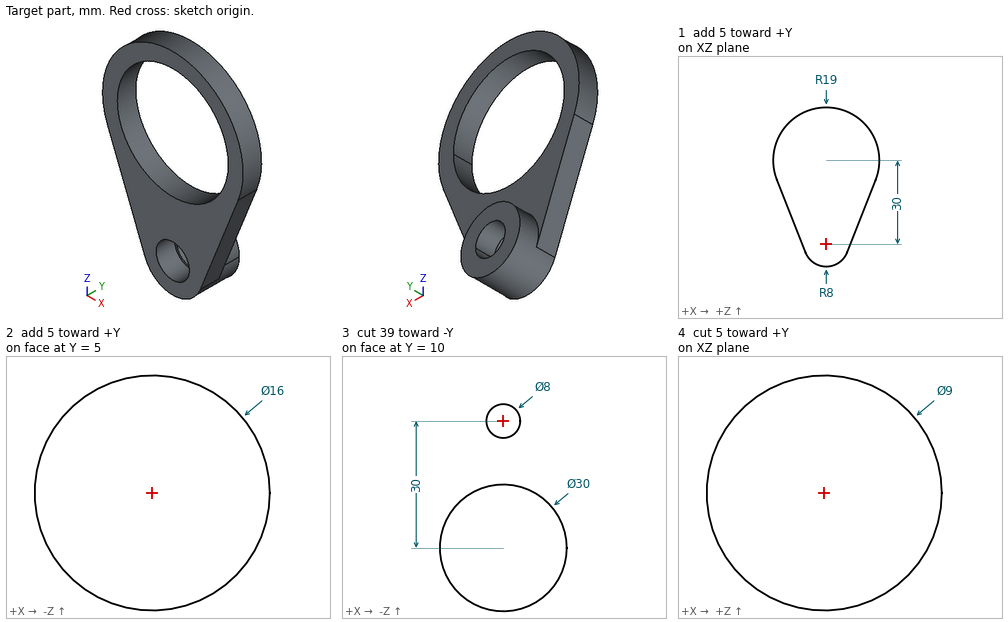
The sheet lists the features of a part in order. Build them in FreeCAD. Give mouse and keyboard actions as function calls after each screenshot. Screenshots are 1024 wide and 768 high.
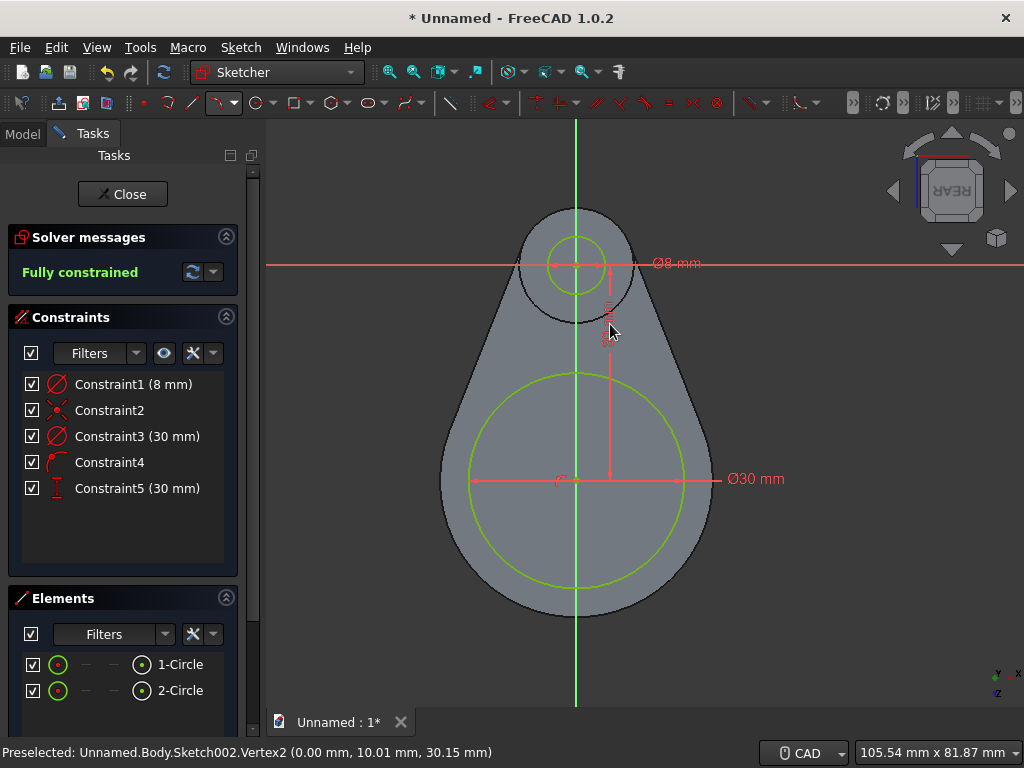
click(123, 194)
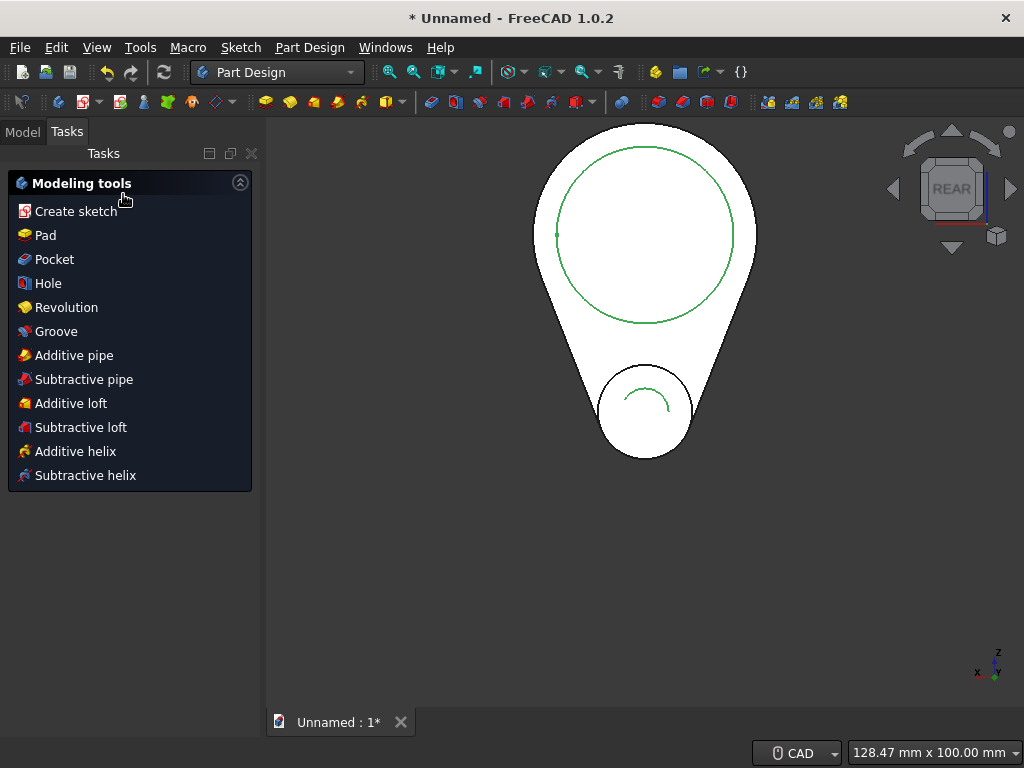
click(432, 102)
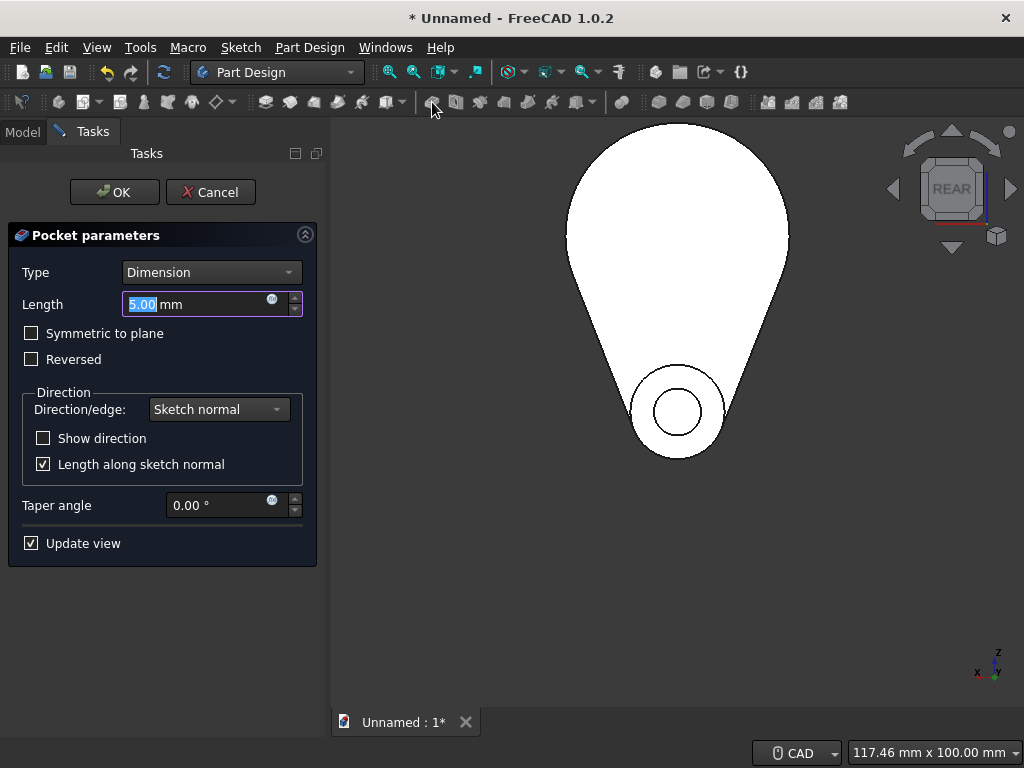
text(39)
key(Tab)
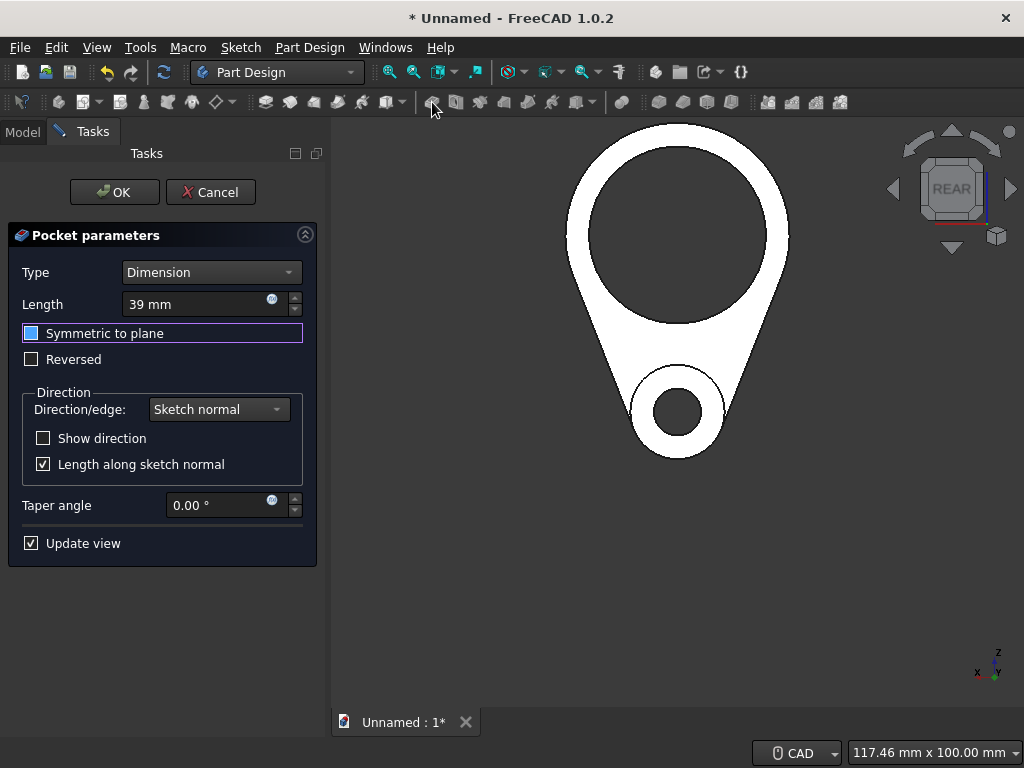
click(115, 192)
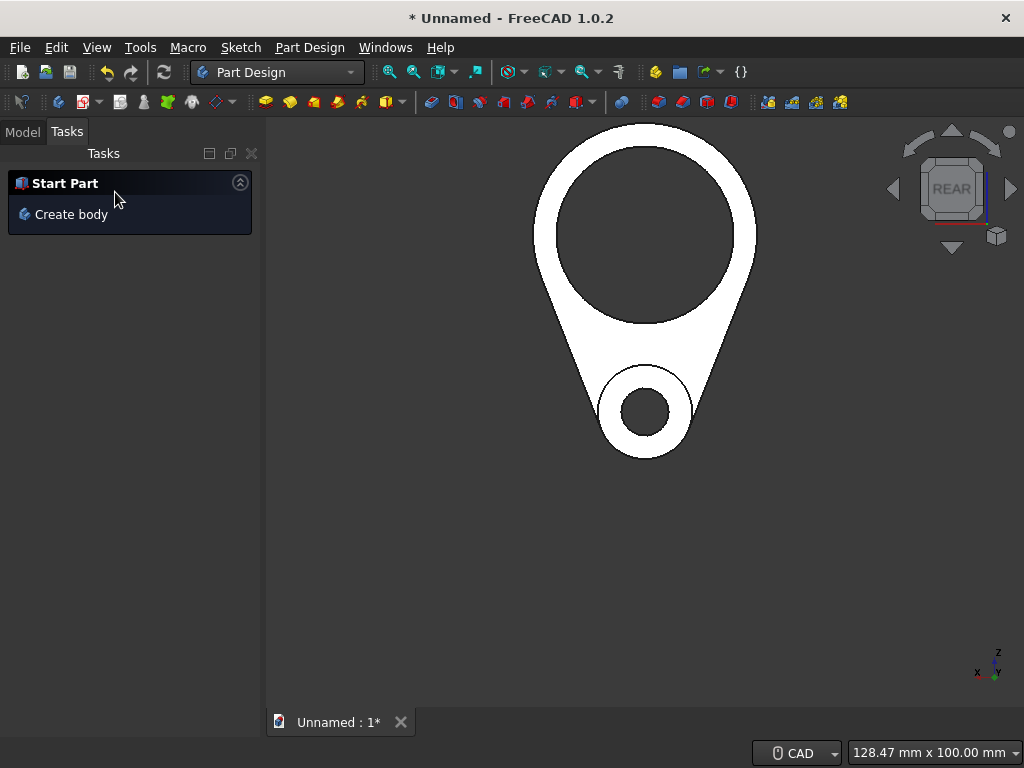
click(84, 102)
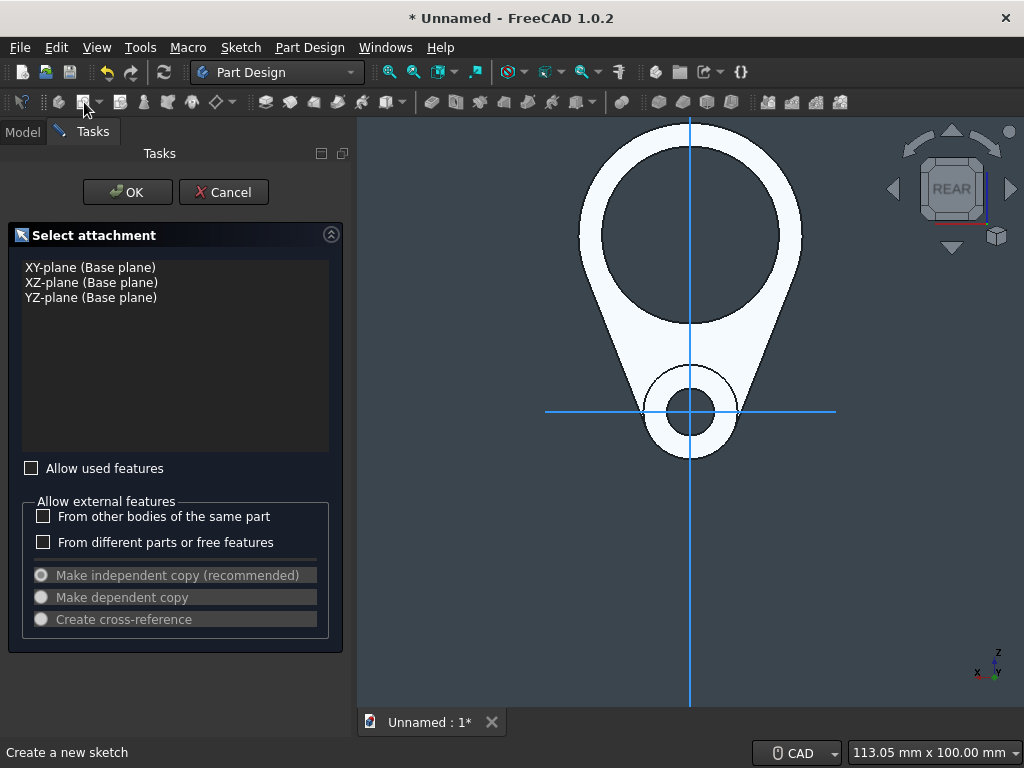
click(82, 282)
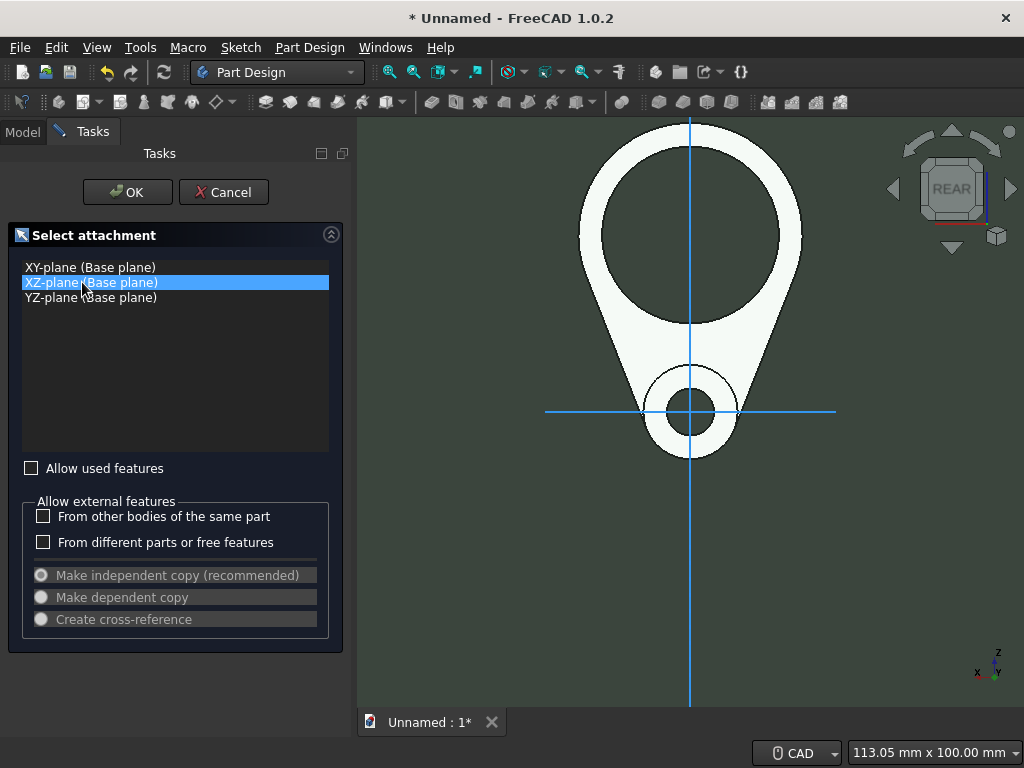
click(128, 192)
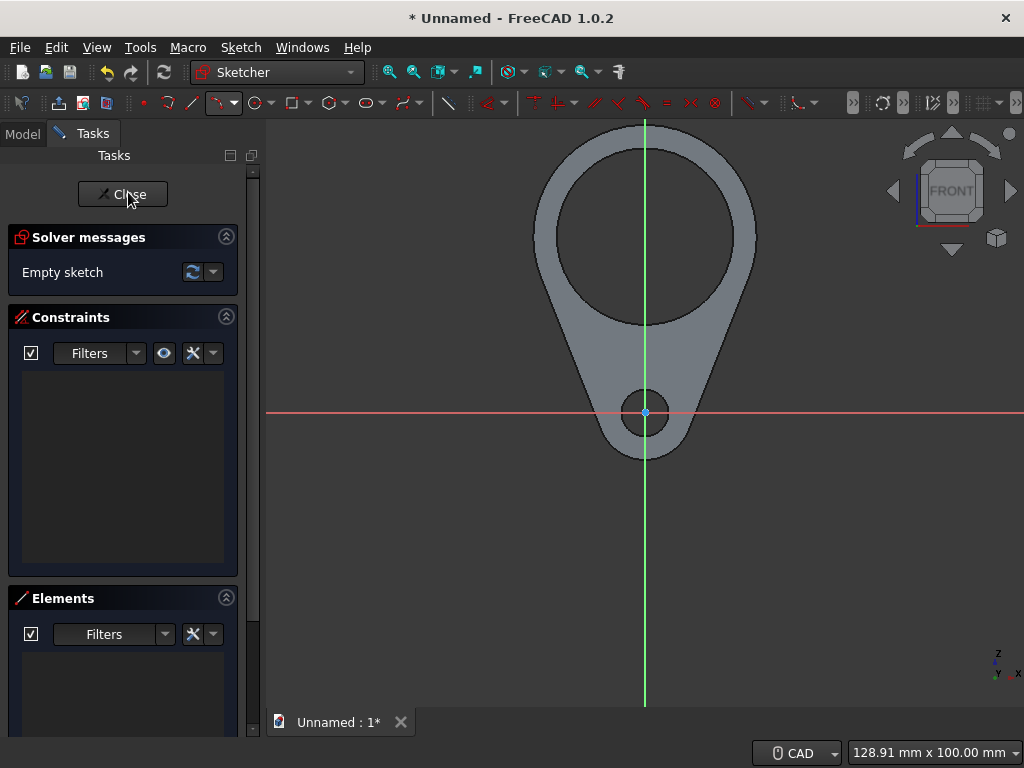
scroll(656, 413, up, 10)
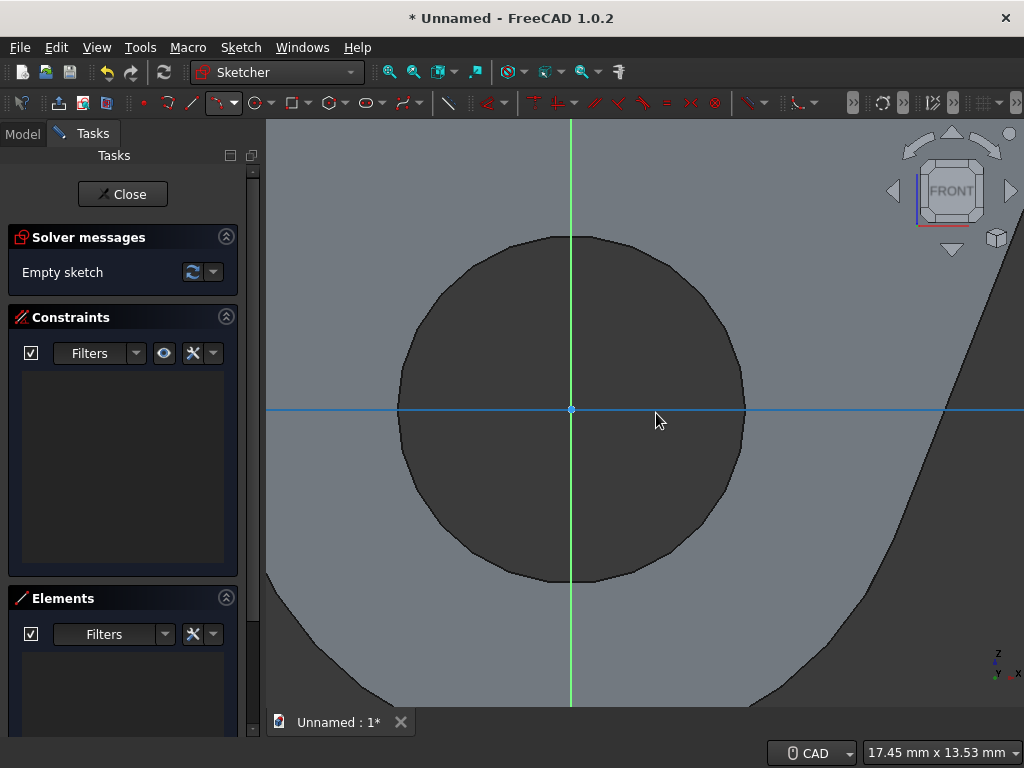
click(256, 104)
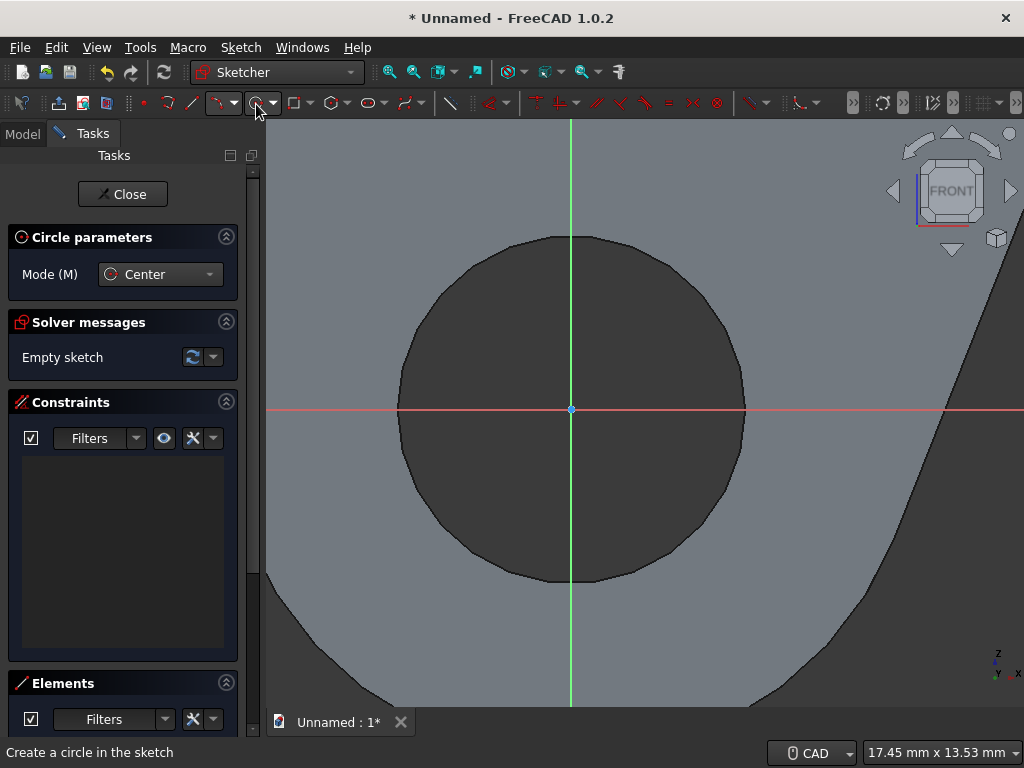
click(571, 410)
move(710, 272)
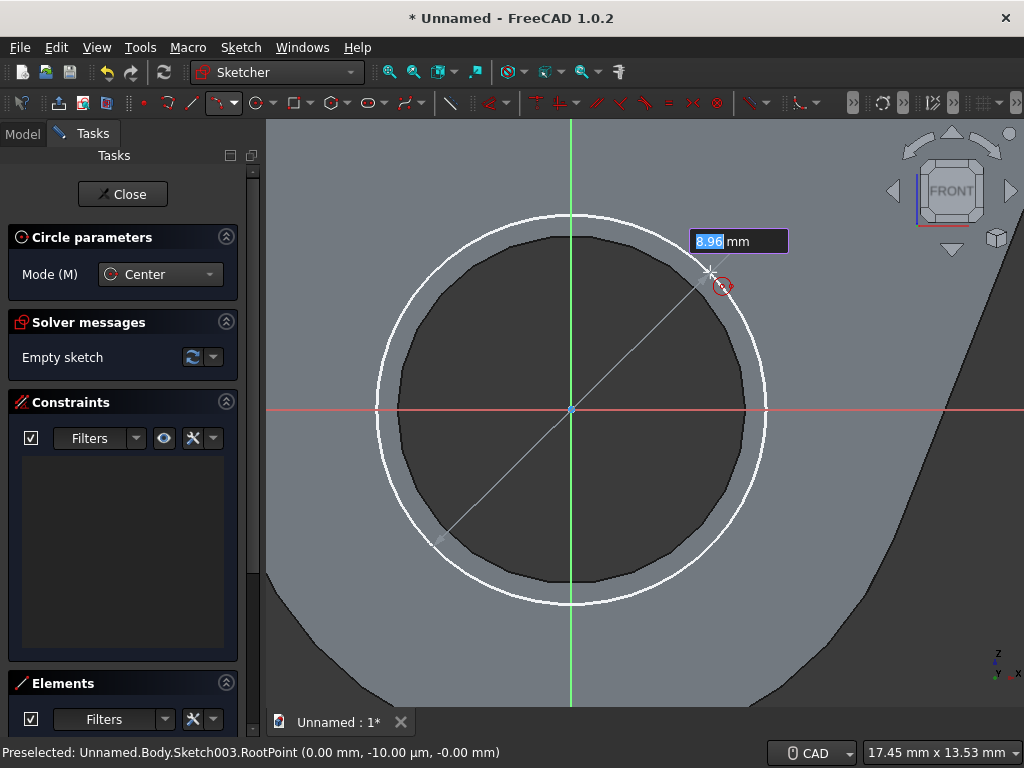
text(9)
key(Return)
key(Escape)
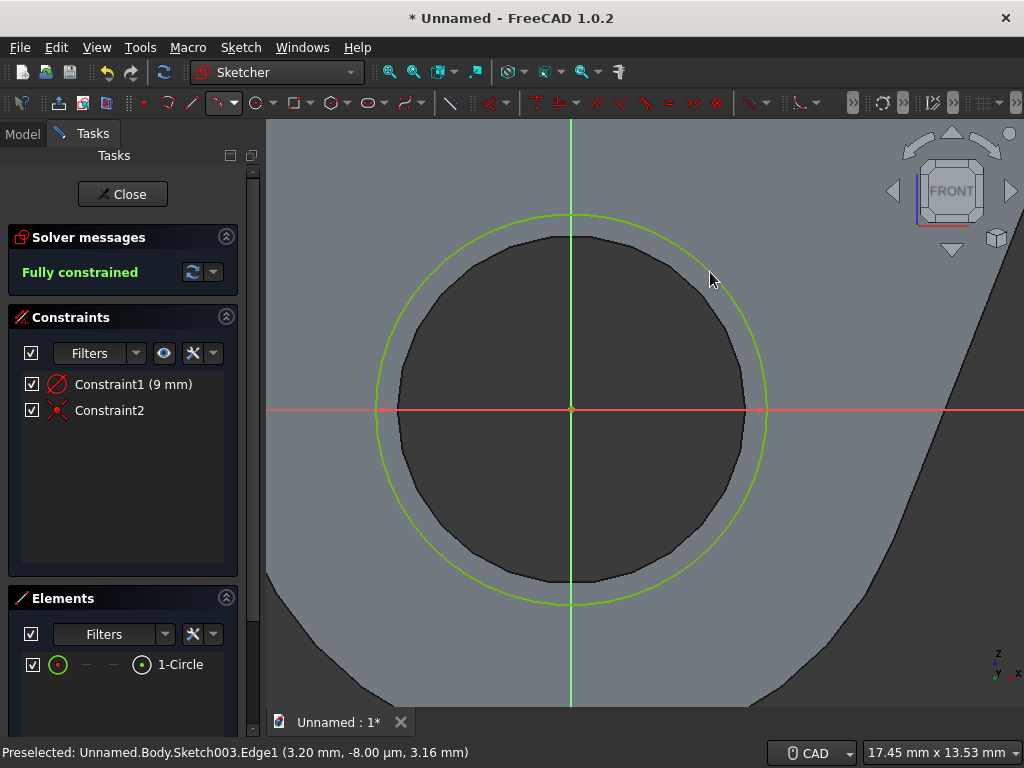
click(123, 194)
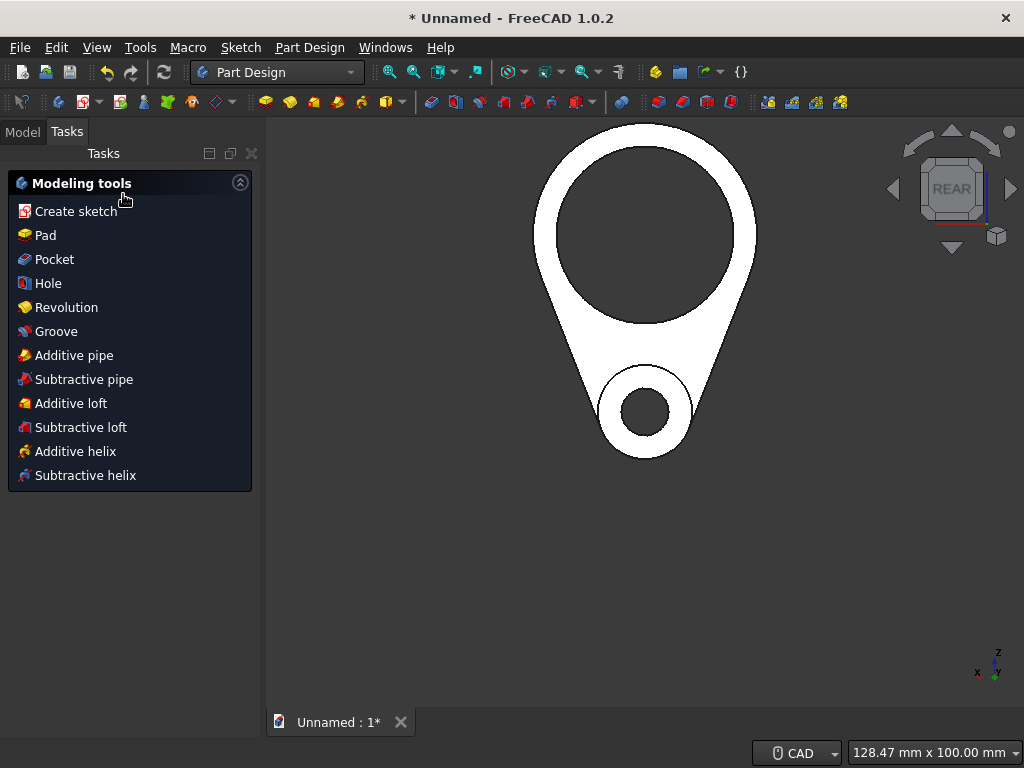
click(432, 102)